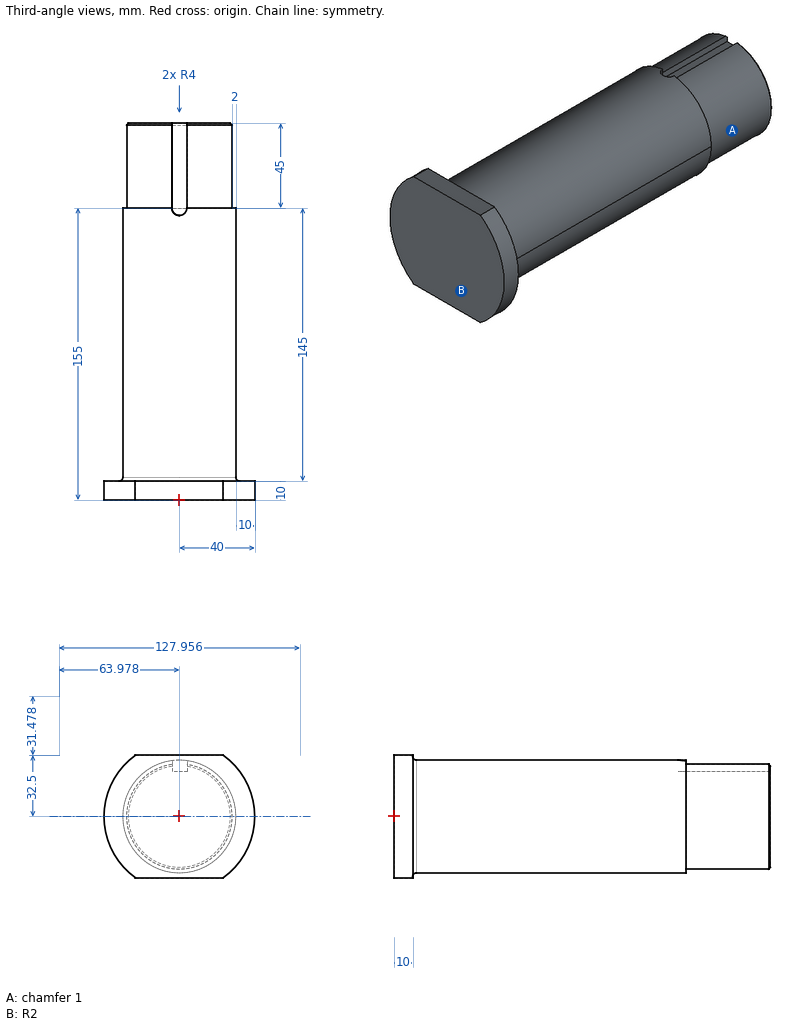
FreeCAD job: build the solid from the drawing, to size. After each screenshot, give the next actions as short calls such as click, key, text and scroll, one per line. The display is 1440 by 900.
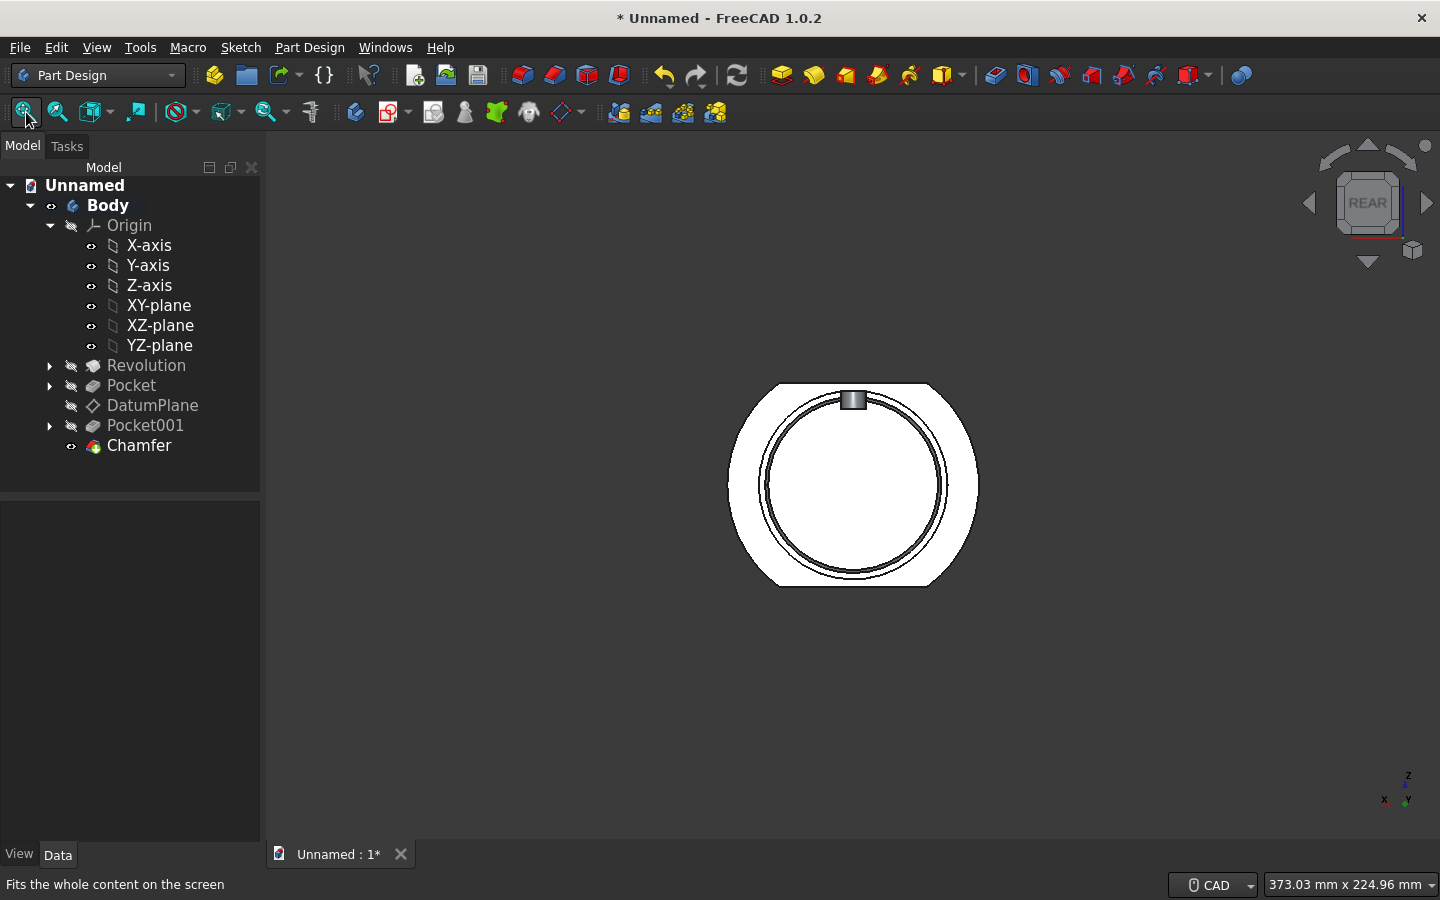
key(6)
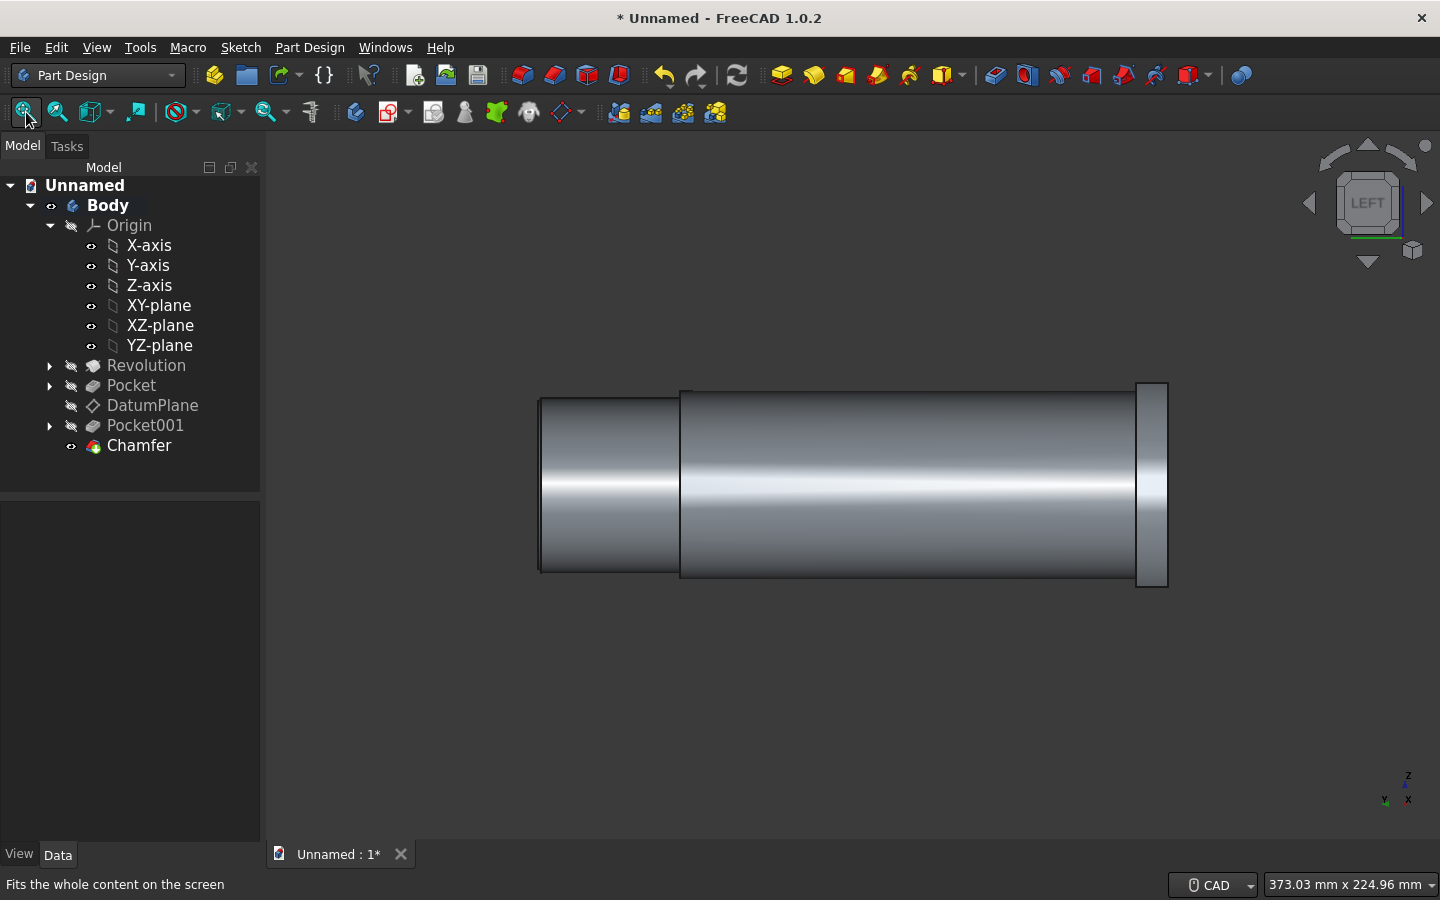
key(v)
key(3)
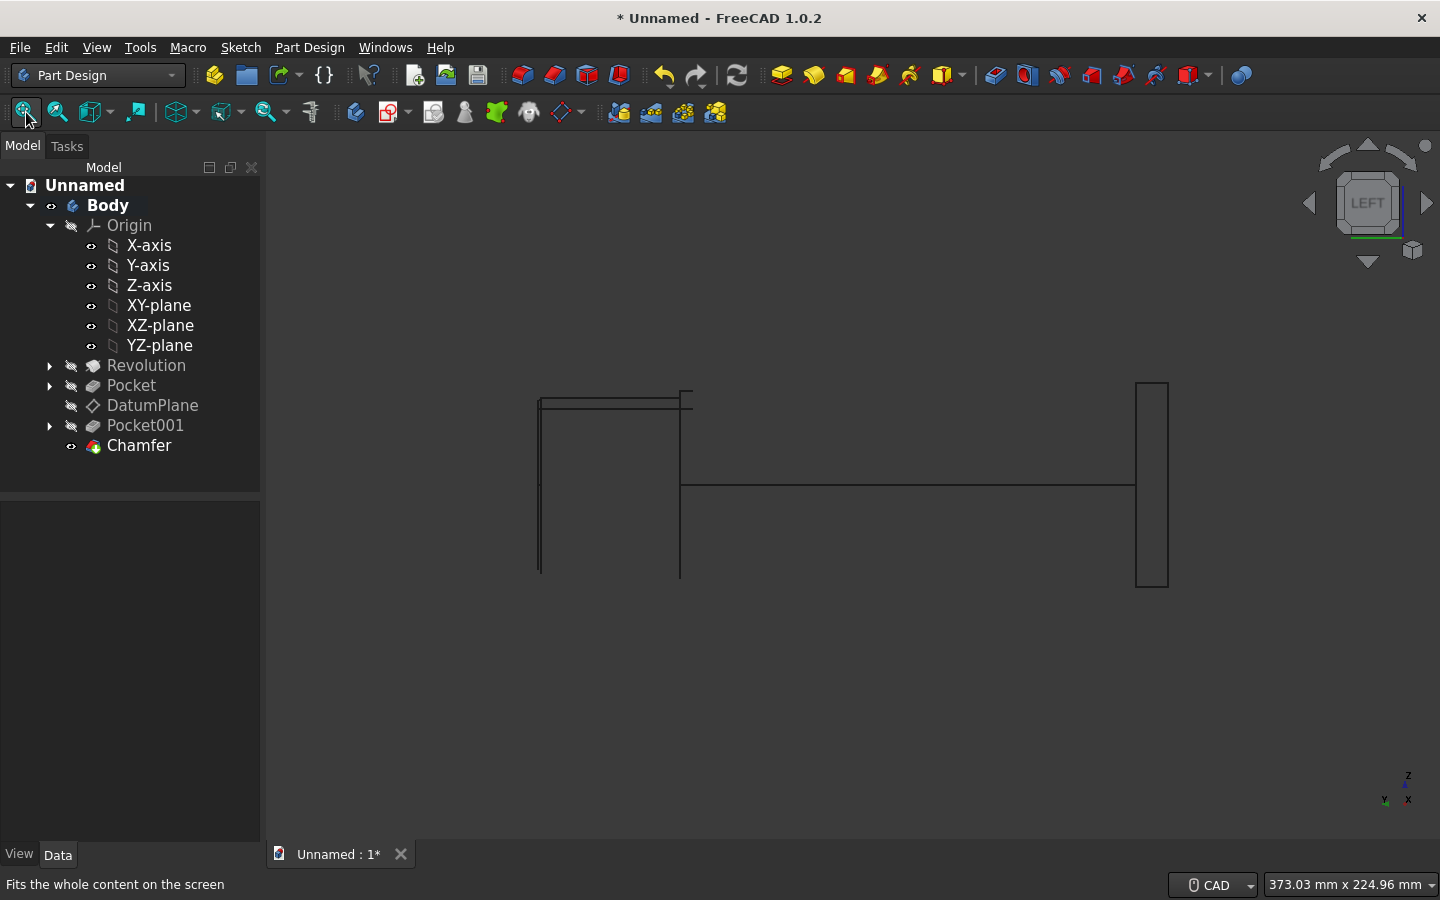
key(0)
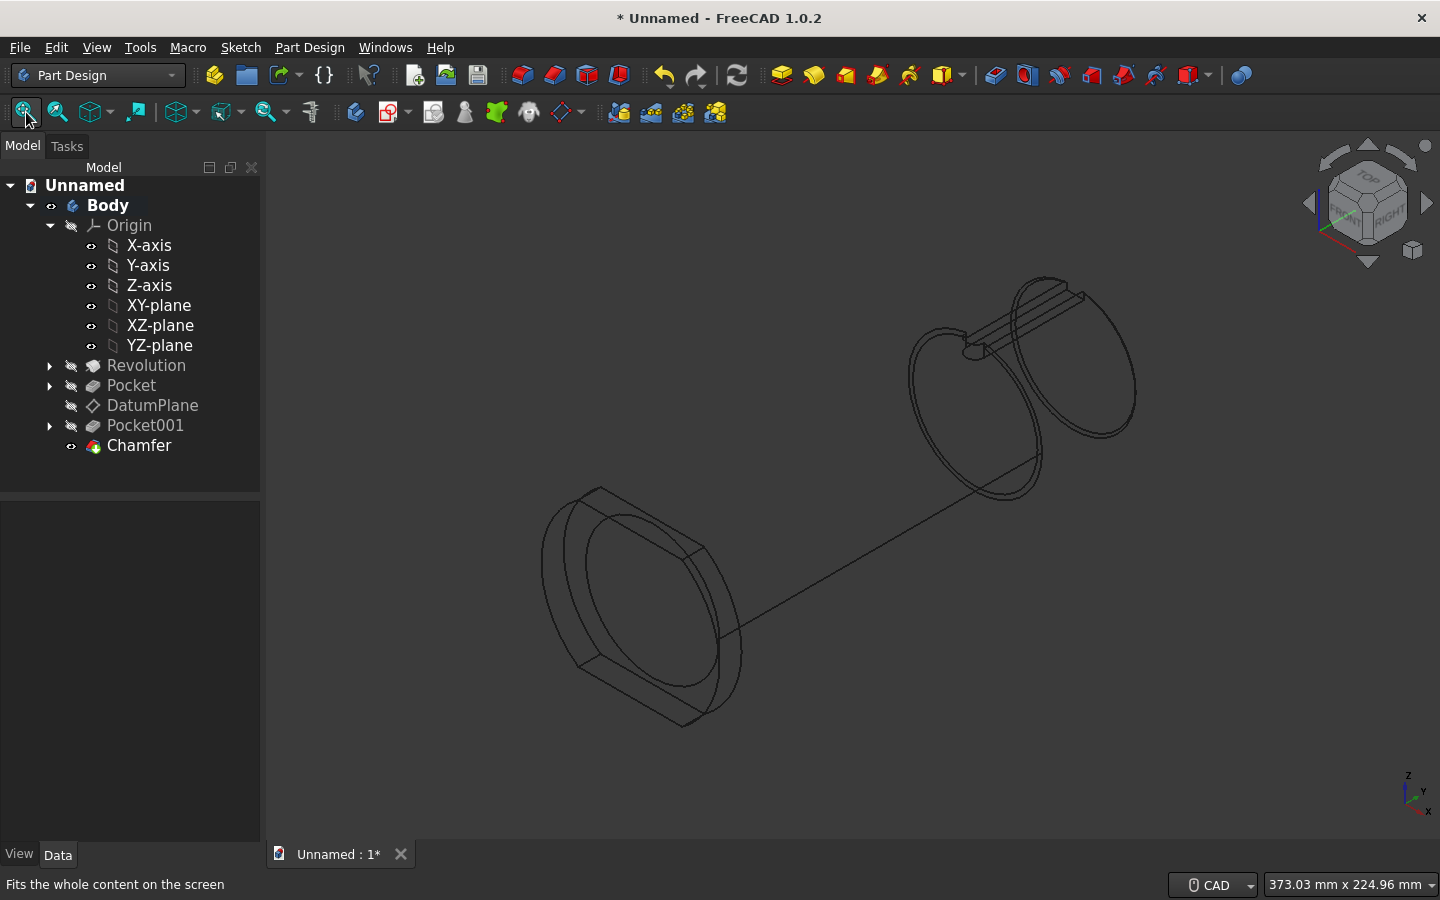
click(586, 561)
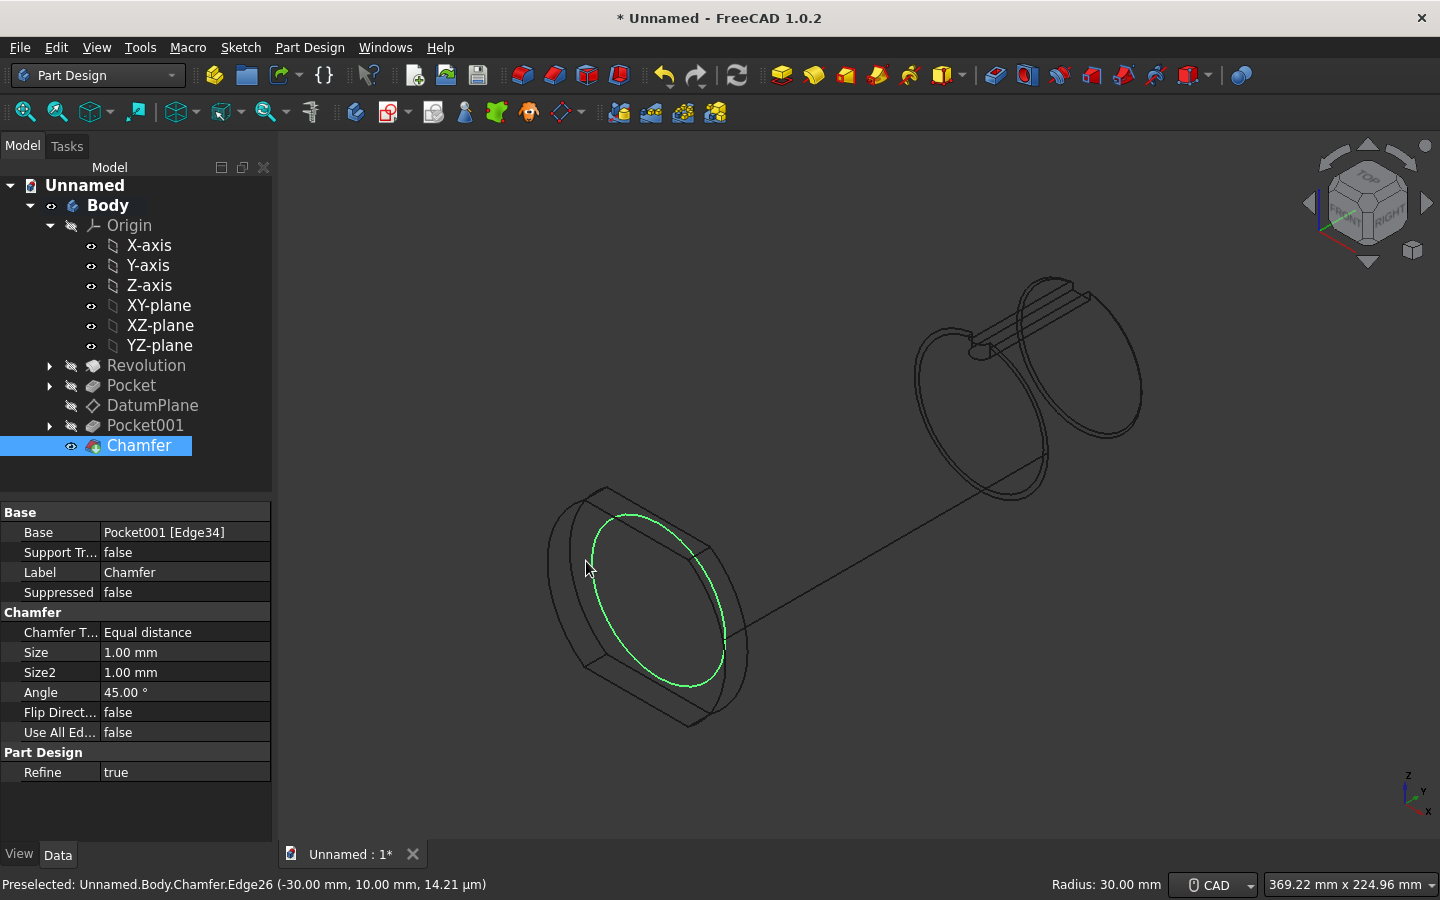
key(v)
key(1)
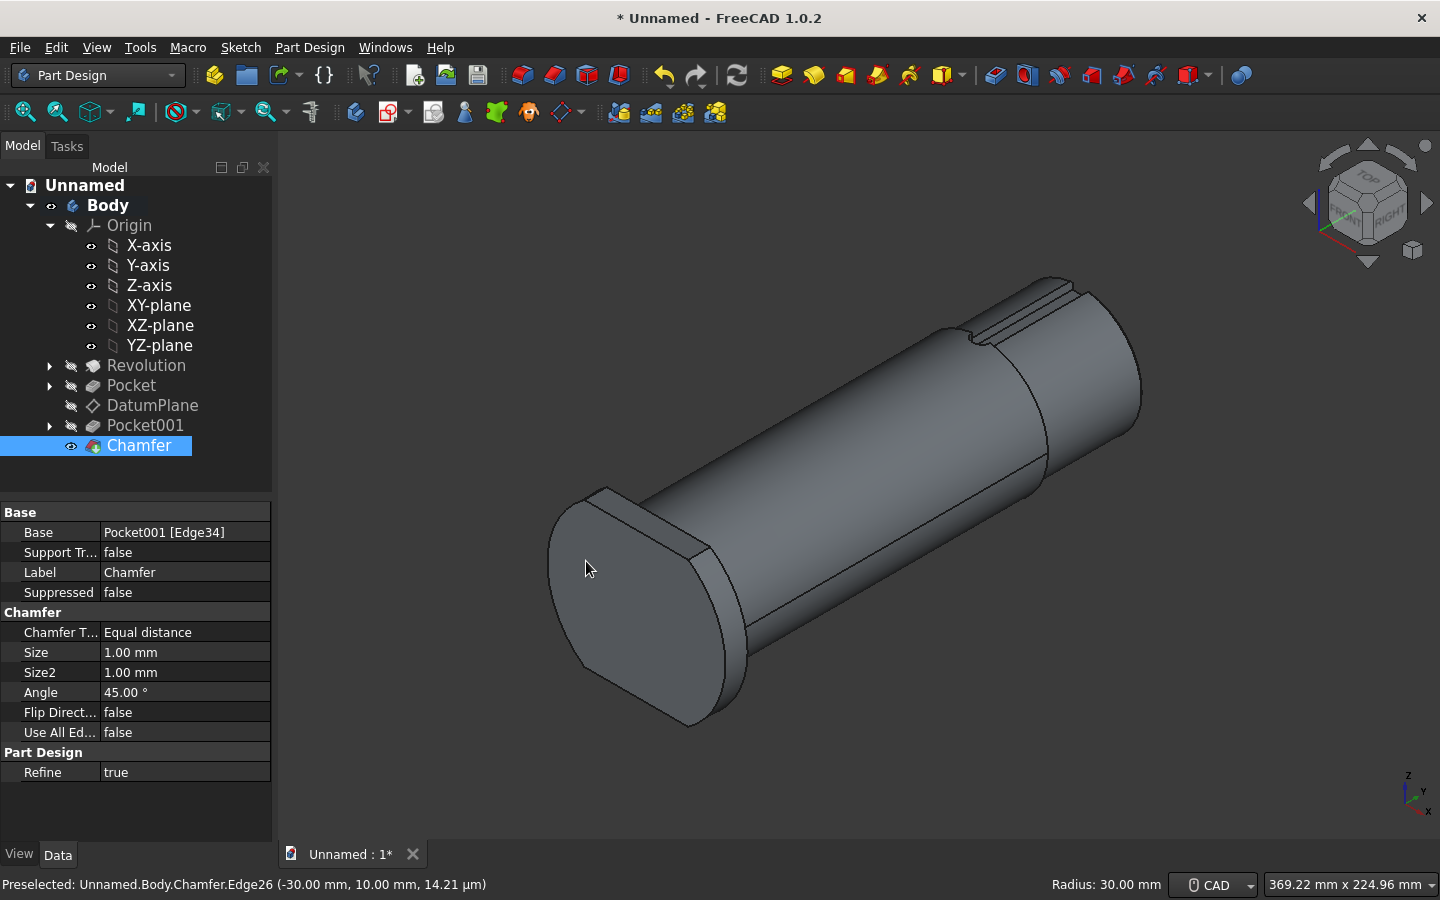
click(524, 76)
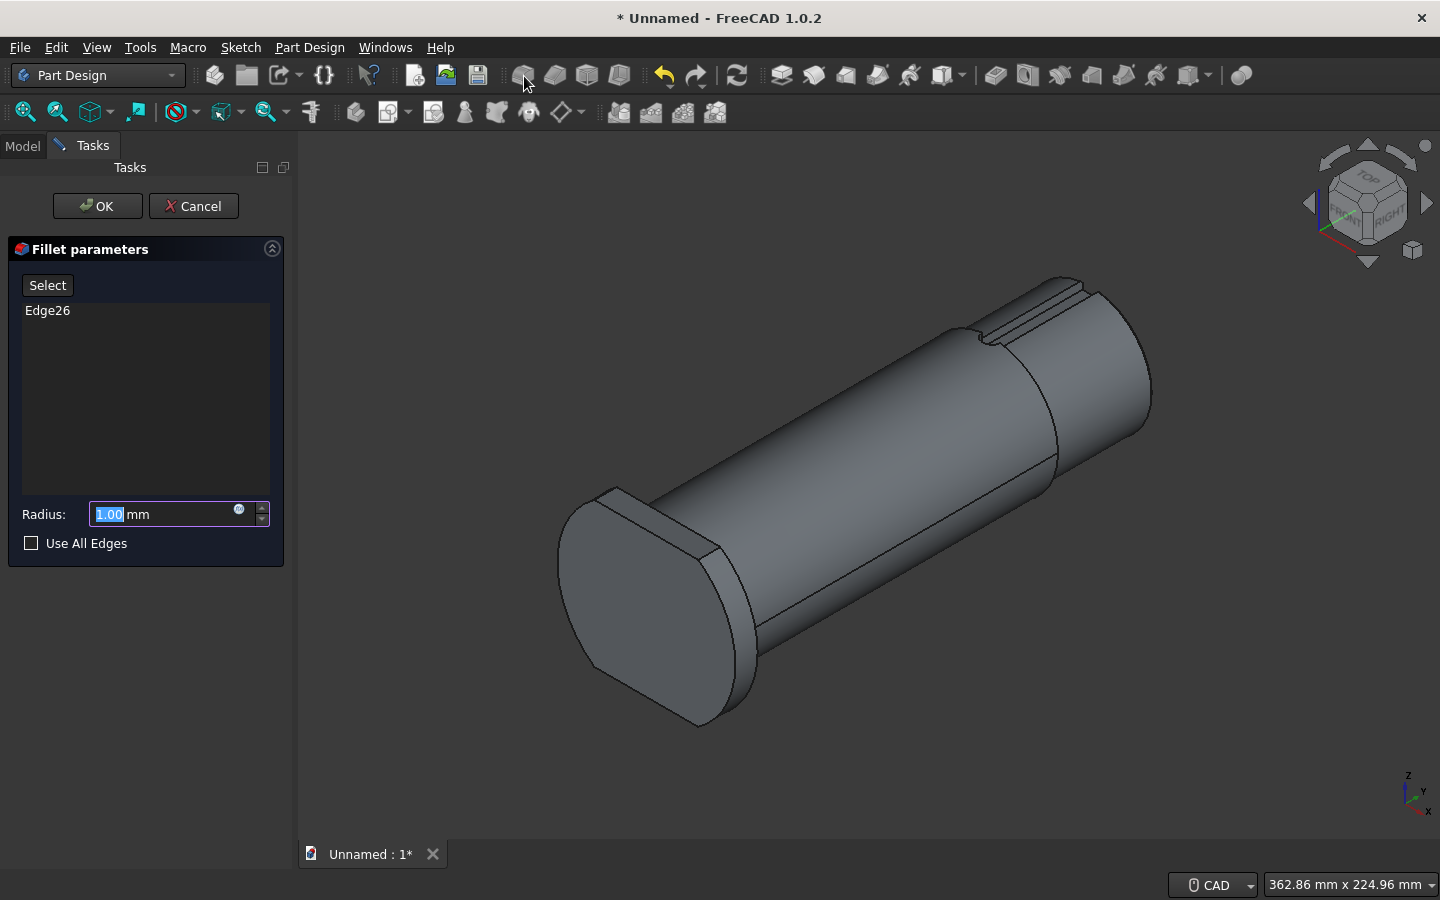
text(2)
key(Tab)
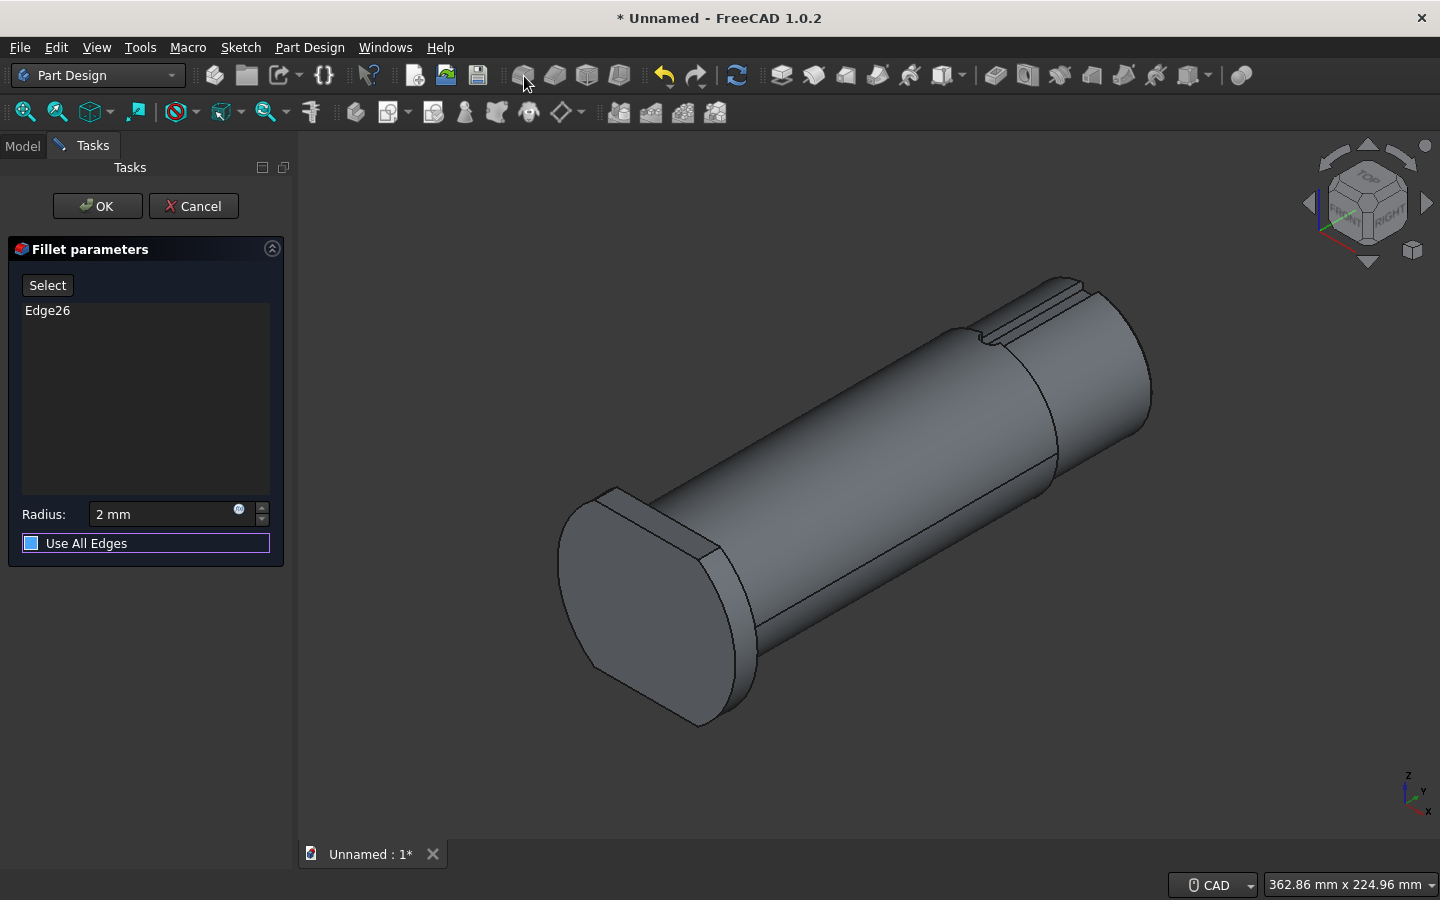
click(98, 206)